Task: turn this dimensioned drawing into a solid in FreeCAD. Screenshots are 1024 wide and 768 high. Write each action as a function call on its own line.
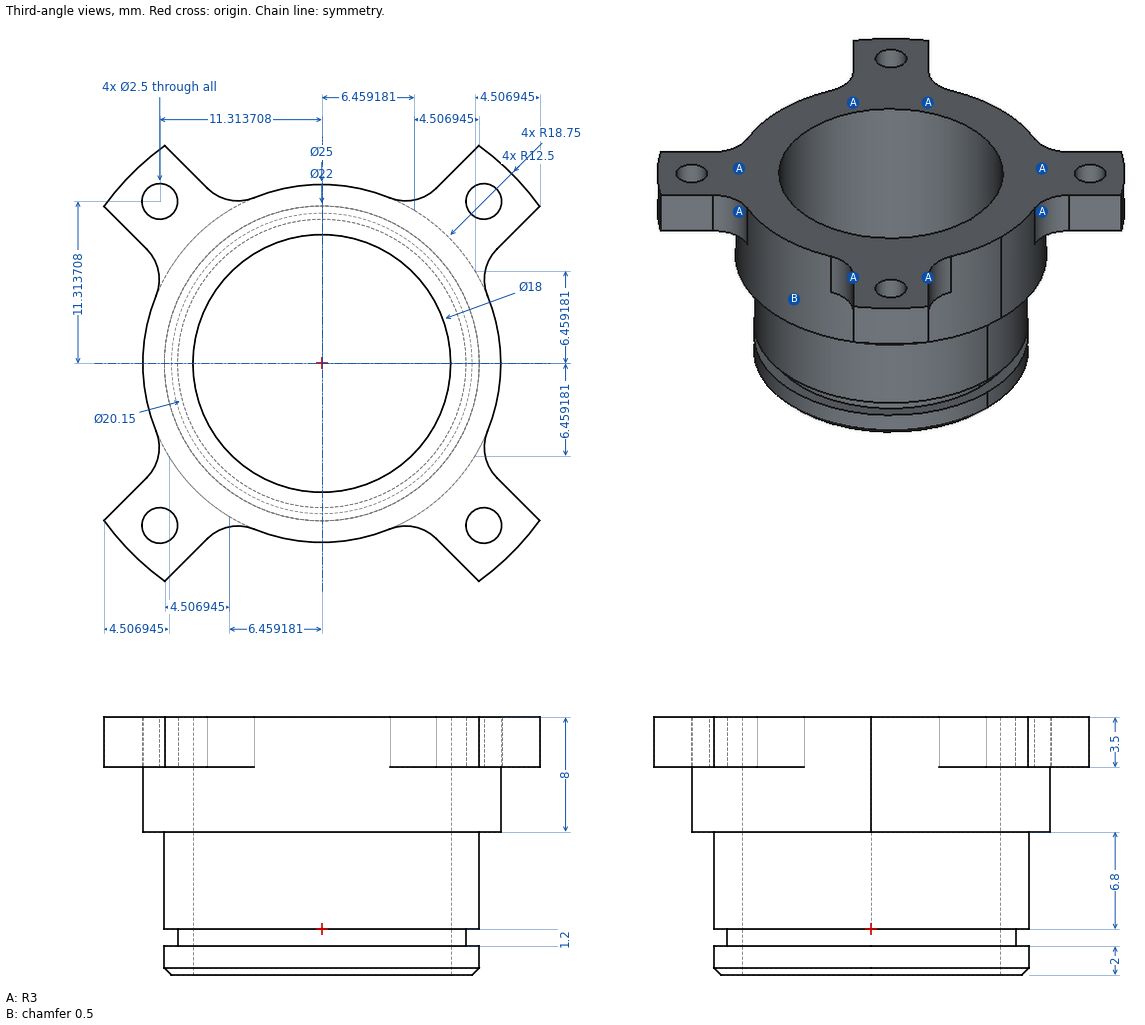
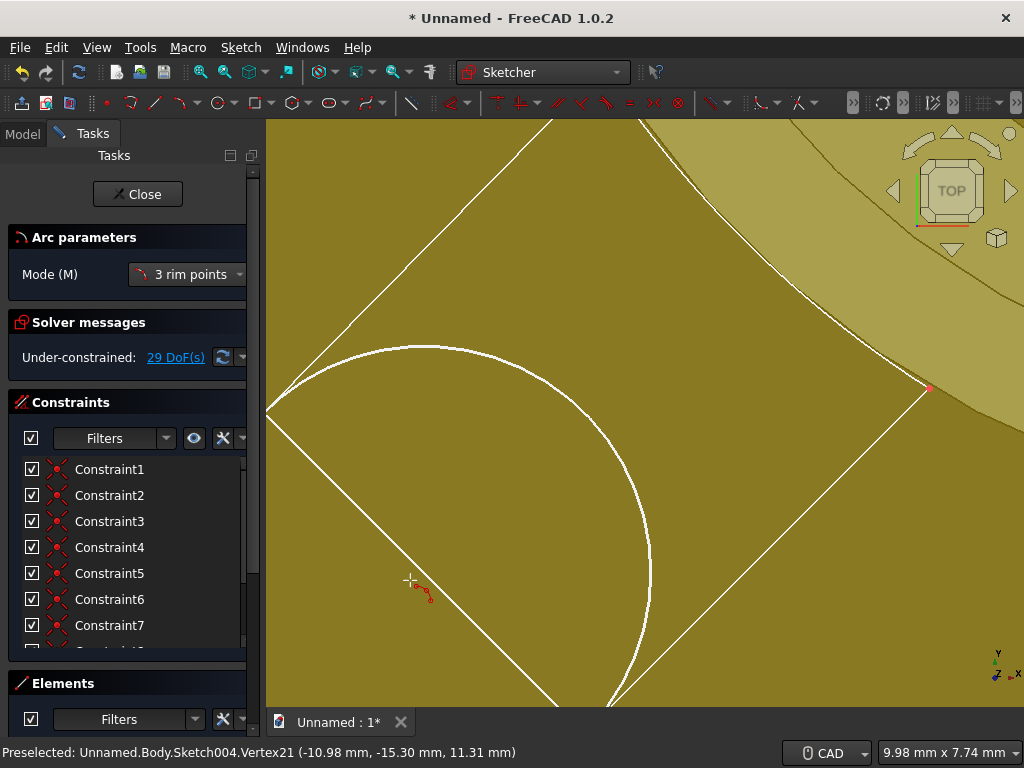
click(411, 578)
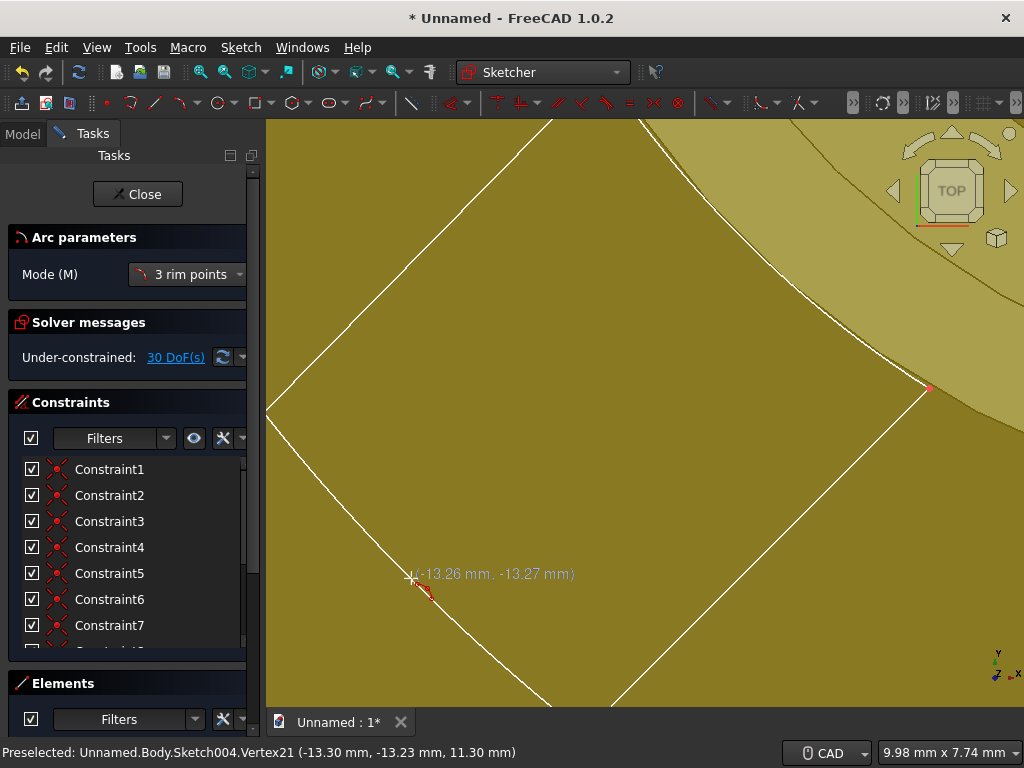
click(156, 104)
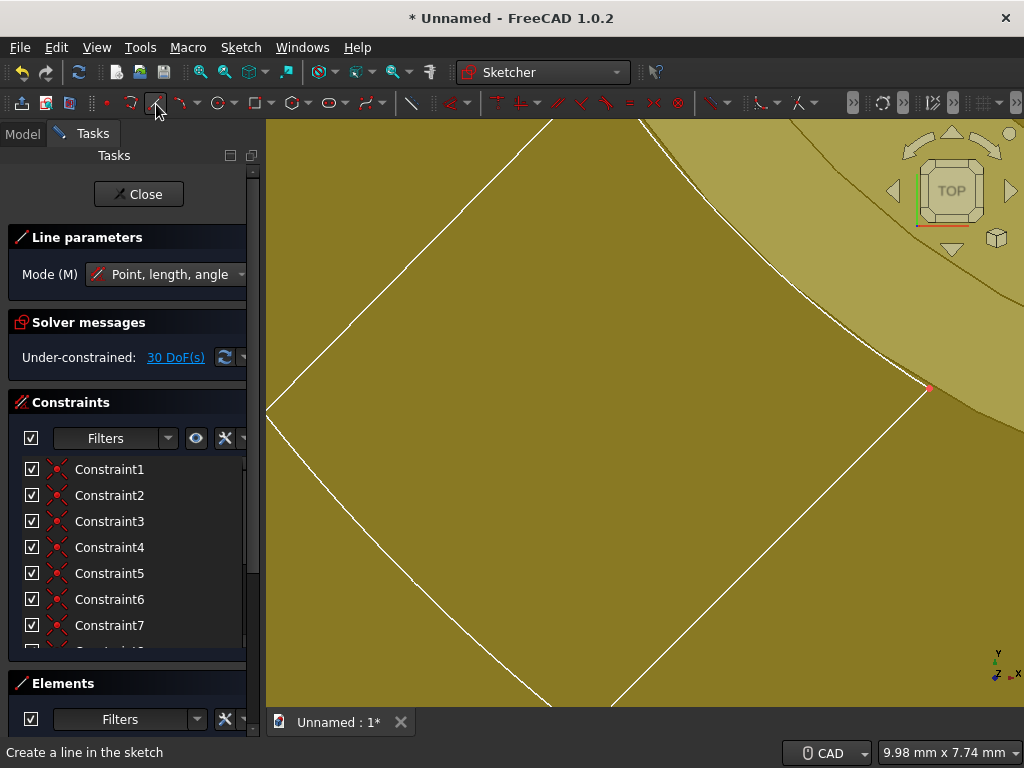
scroll(410, 580, down, 9)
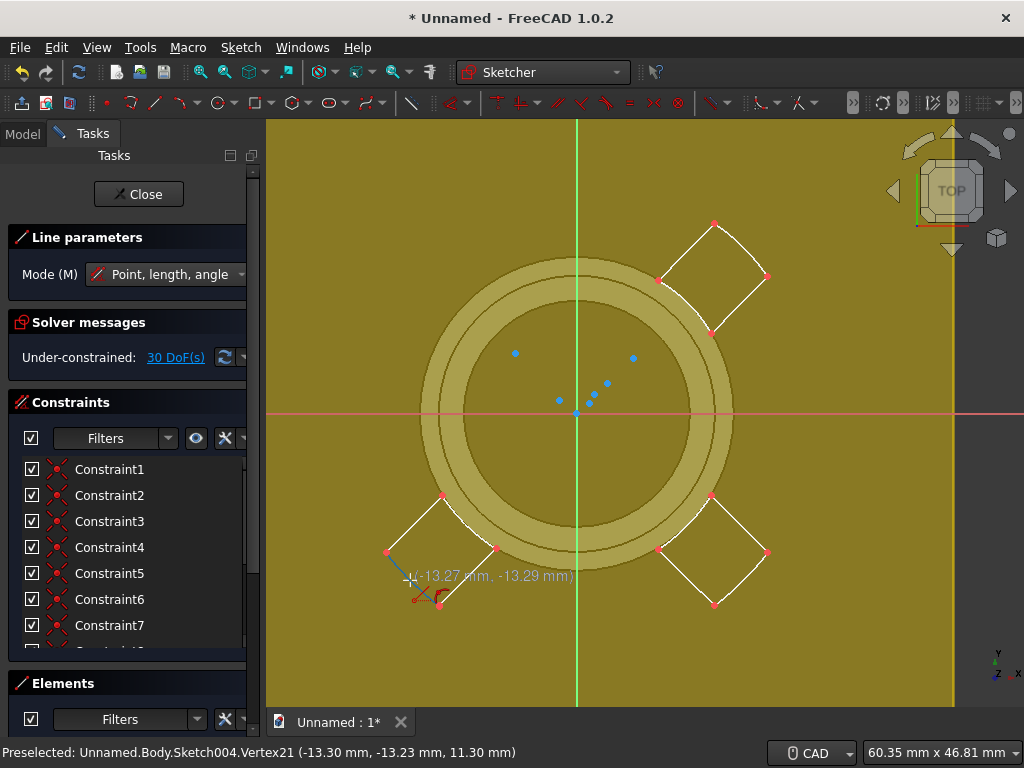
click(386, 276)
click(442, 333)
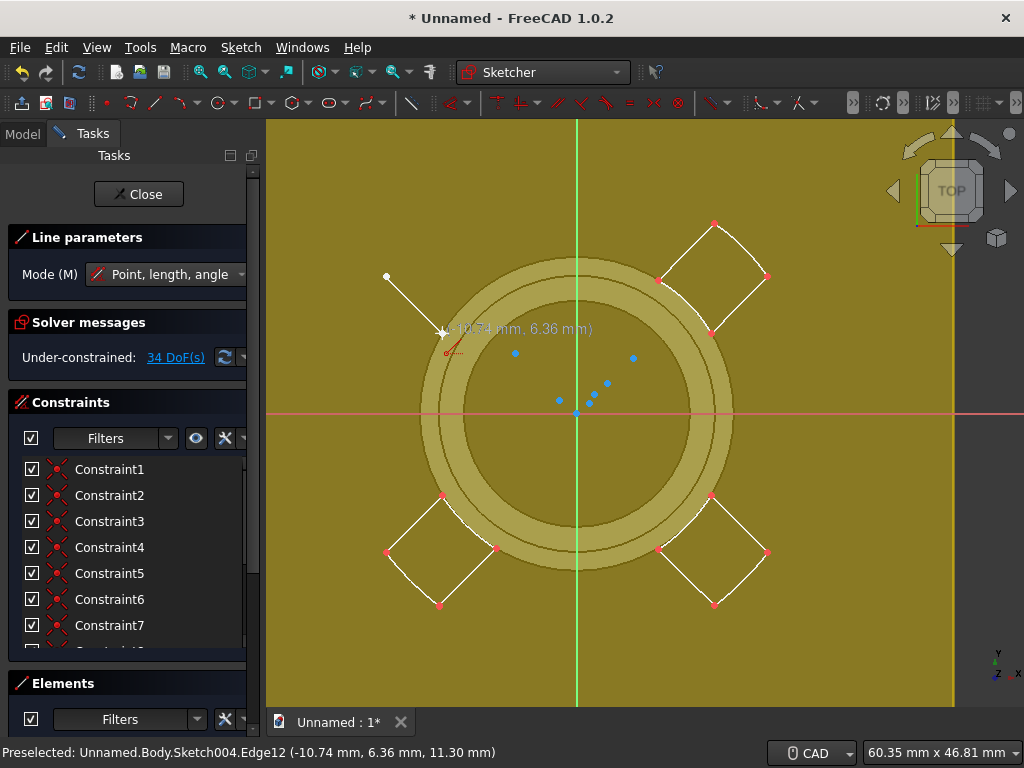
click(496, 279)
click(439, 223)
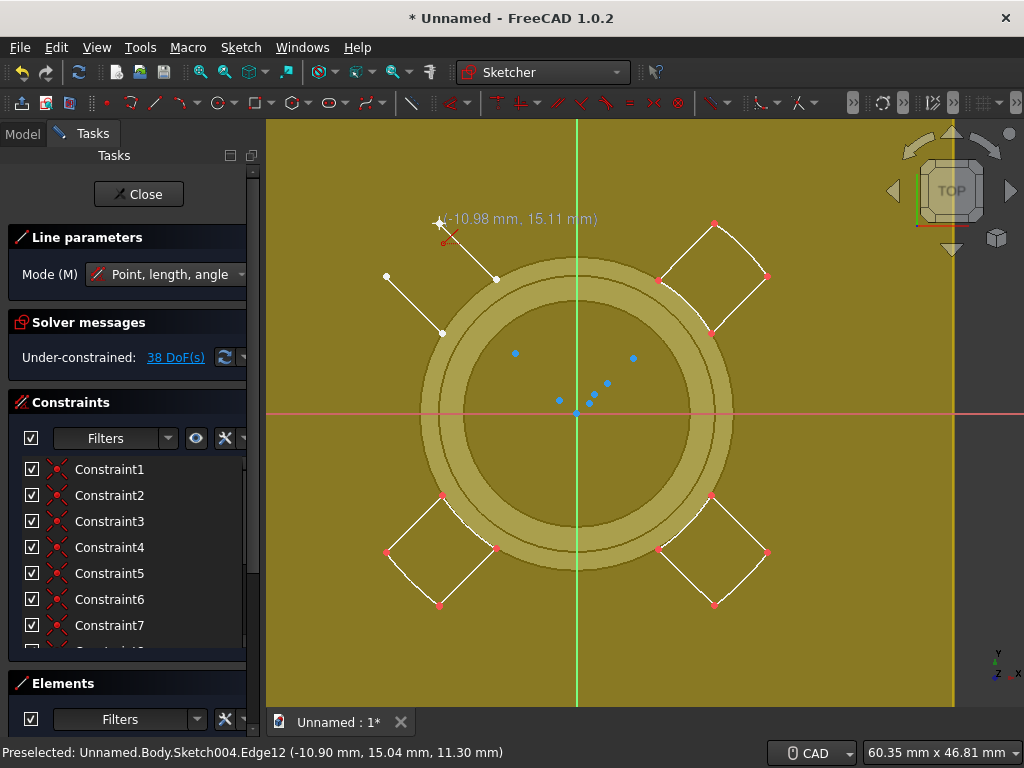
click(180, 104)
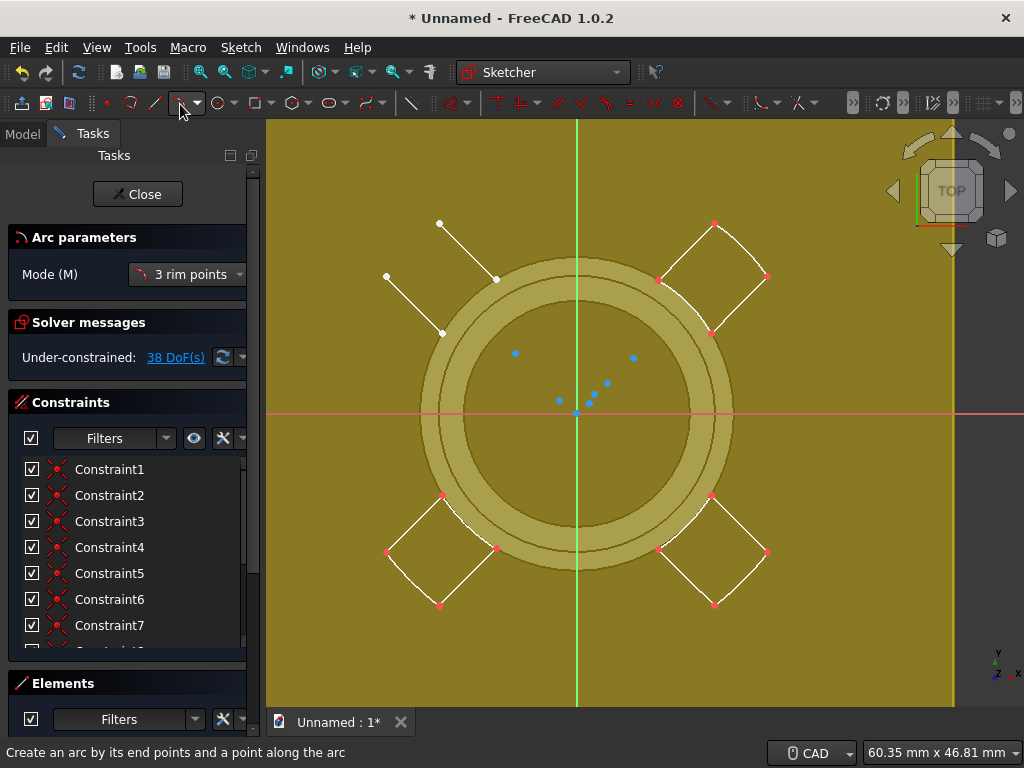
click(442, 334)
click(496, 280)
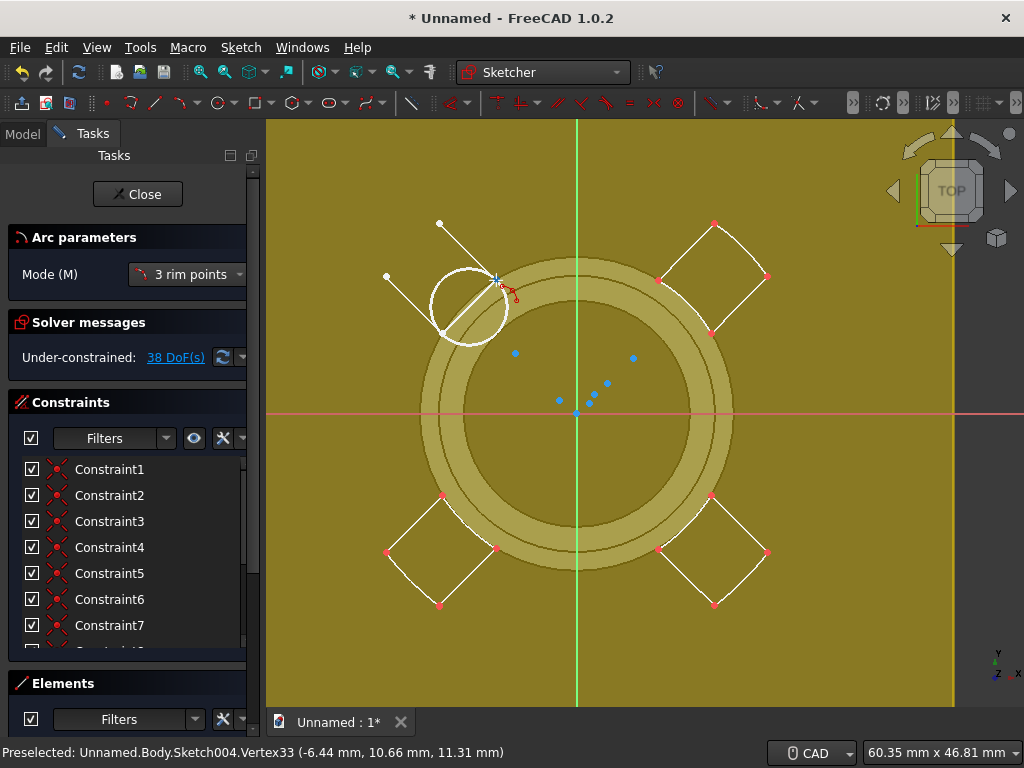
scroll(466, 303, up, 7)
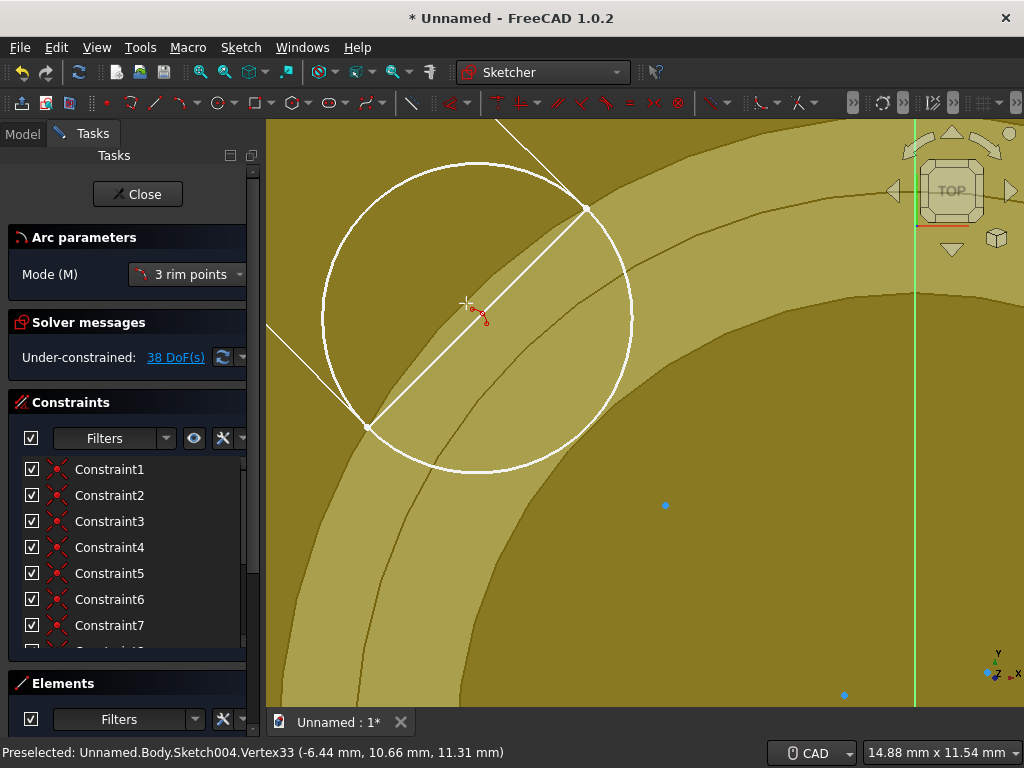
click(465, 301)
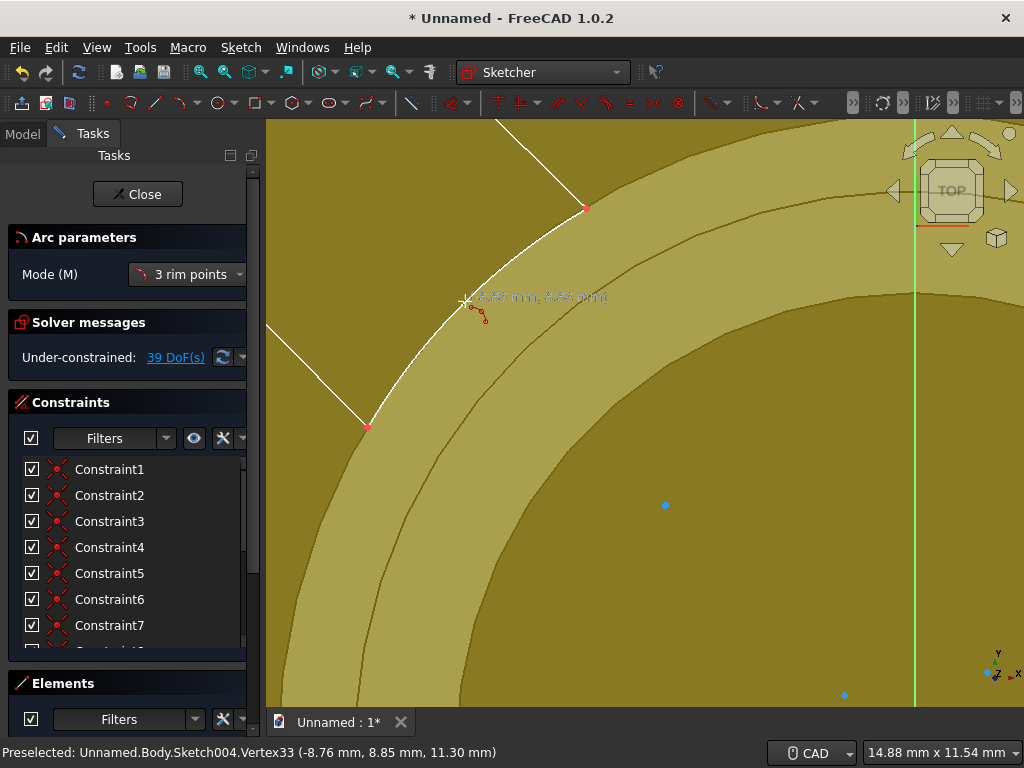
scroll(466, 302, down, 7)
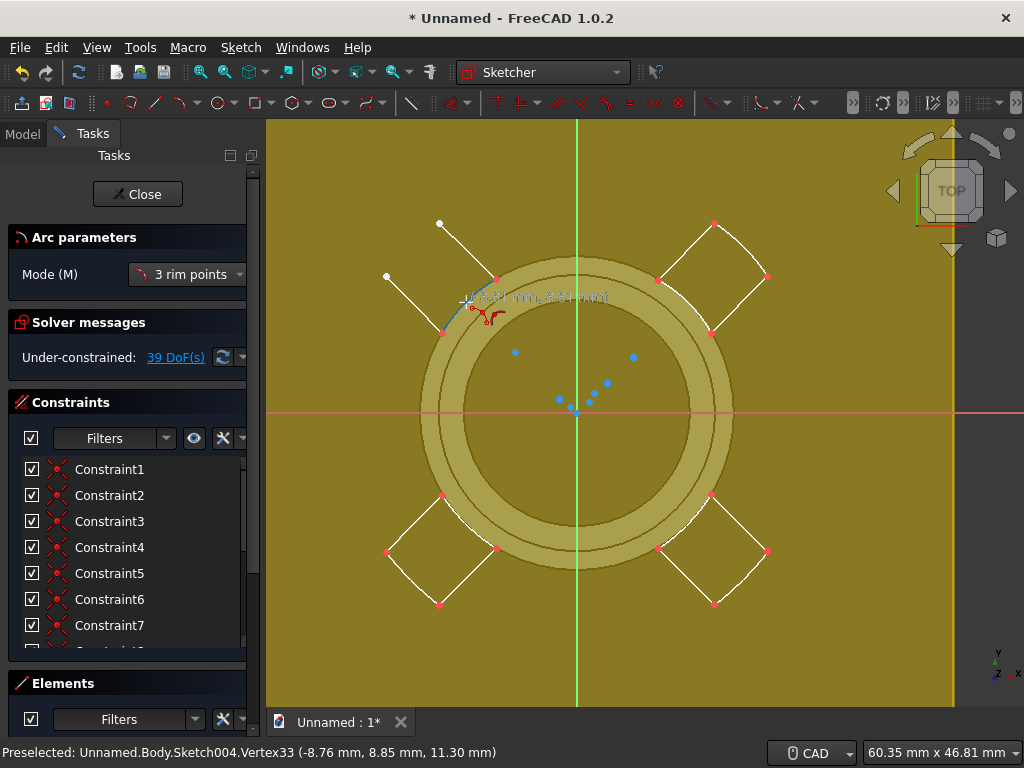
click(439, 223)
click(386, 276)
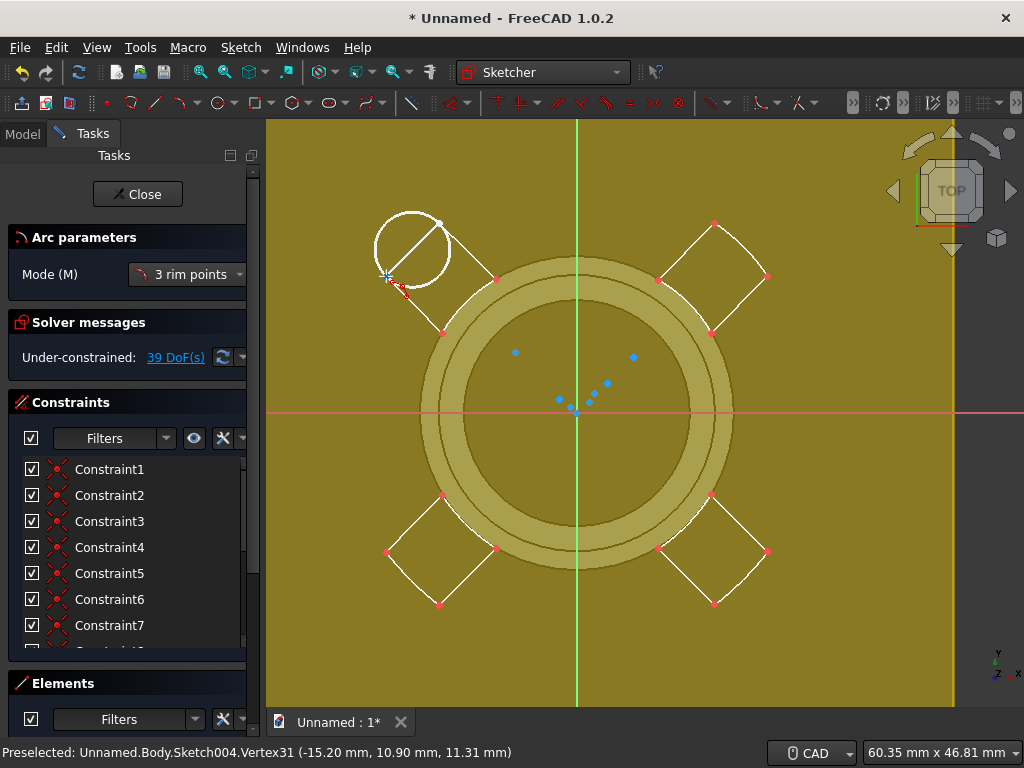
scroll(410, 247, up, 9)